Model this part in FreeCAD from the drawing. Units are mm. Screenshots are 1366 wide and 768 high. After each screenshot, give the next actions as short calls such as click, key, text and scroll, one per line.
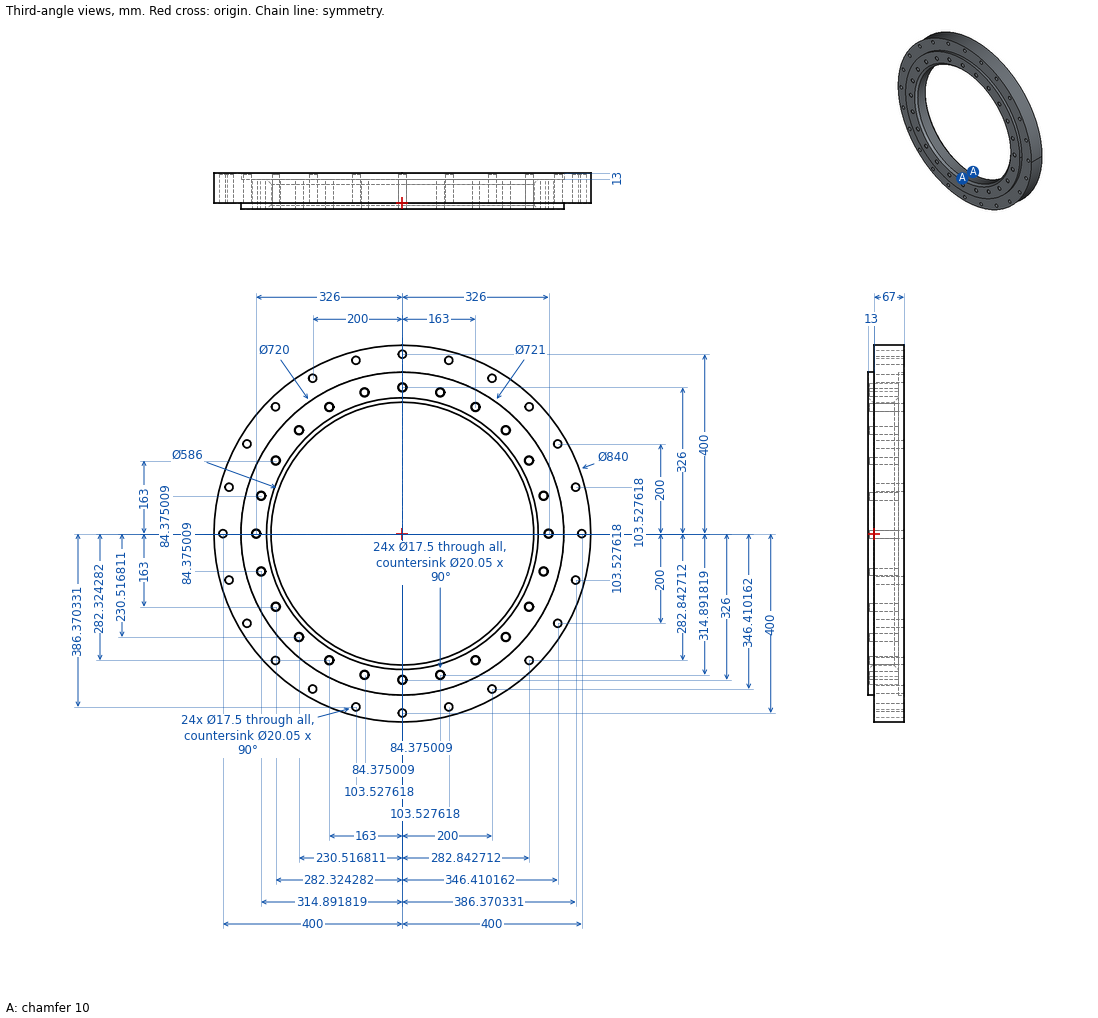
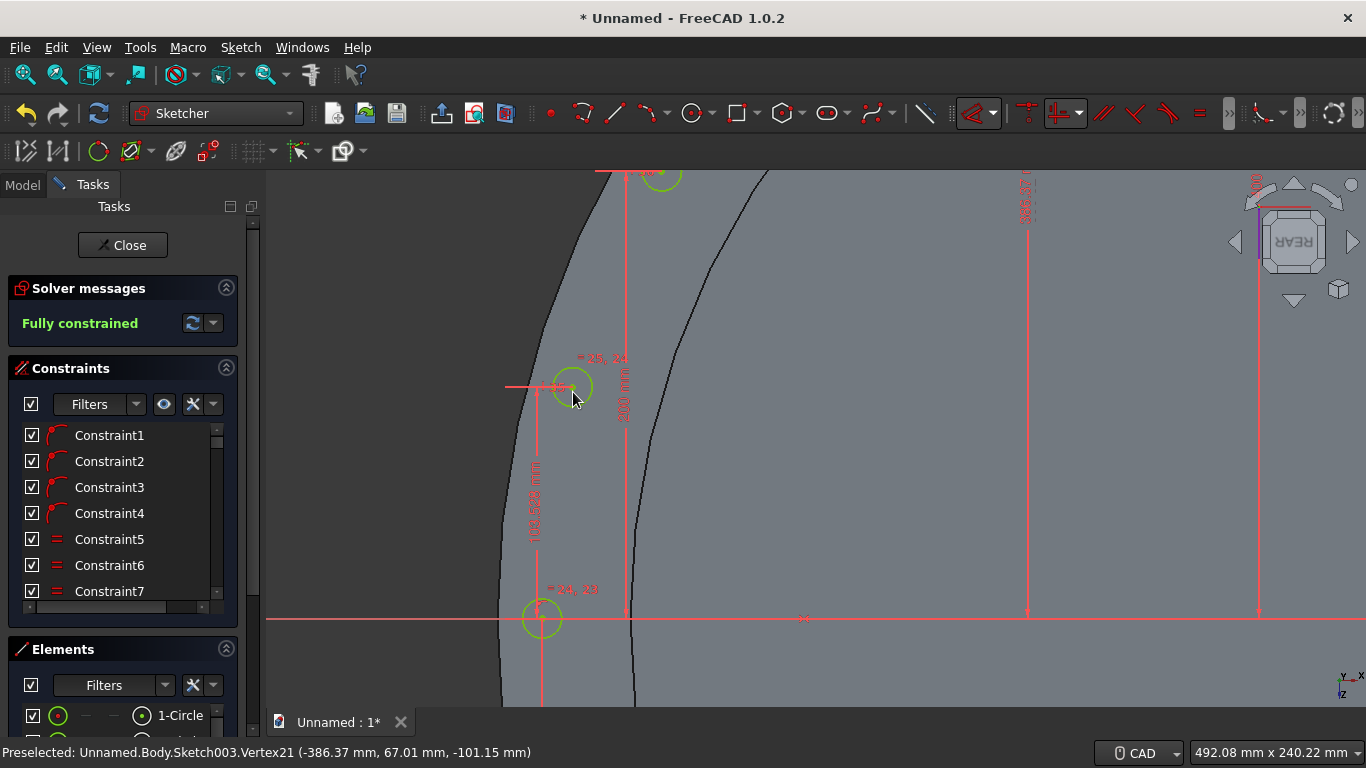
click(123, 245)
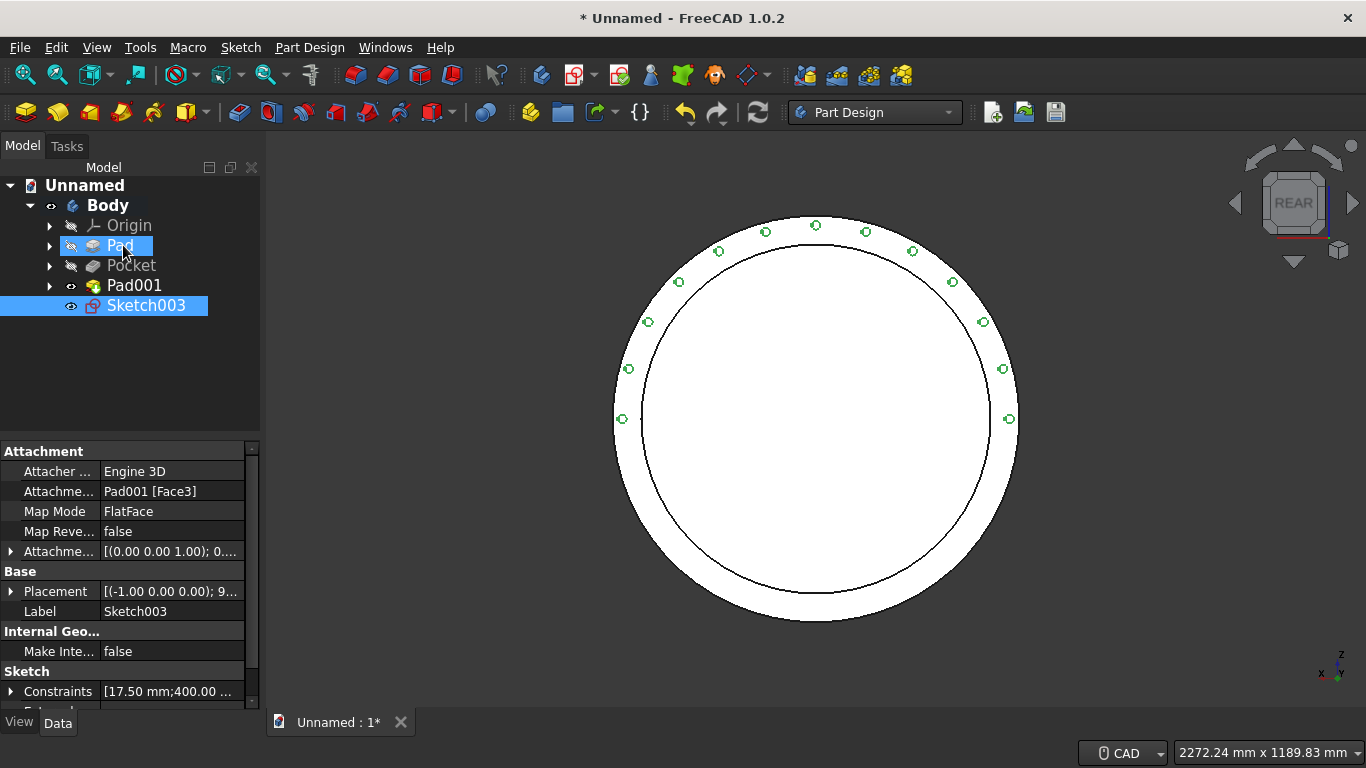
click(272, 112)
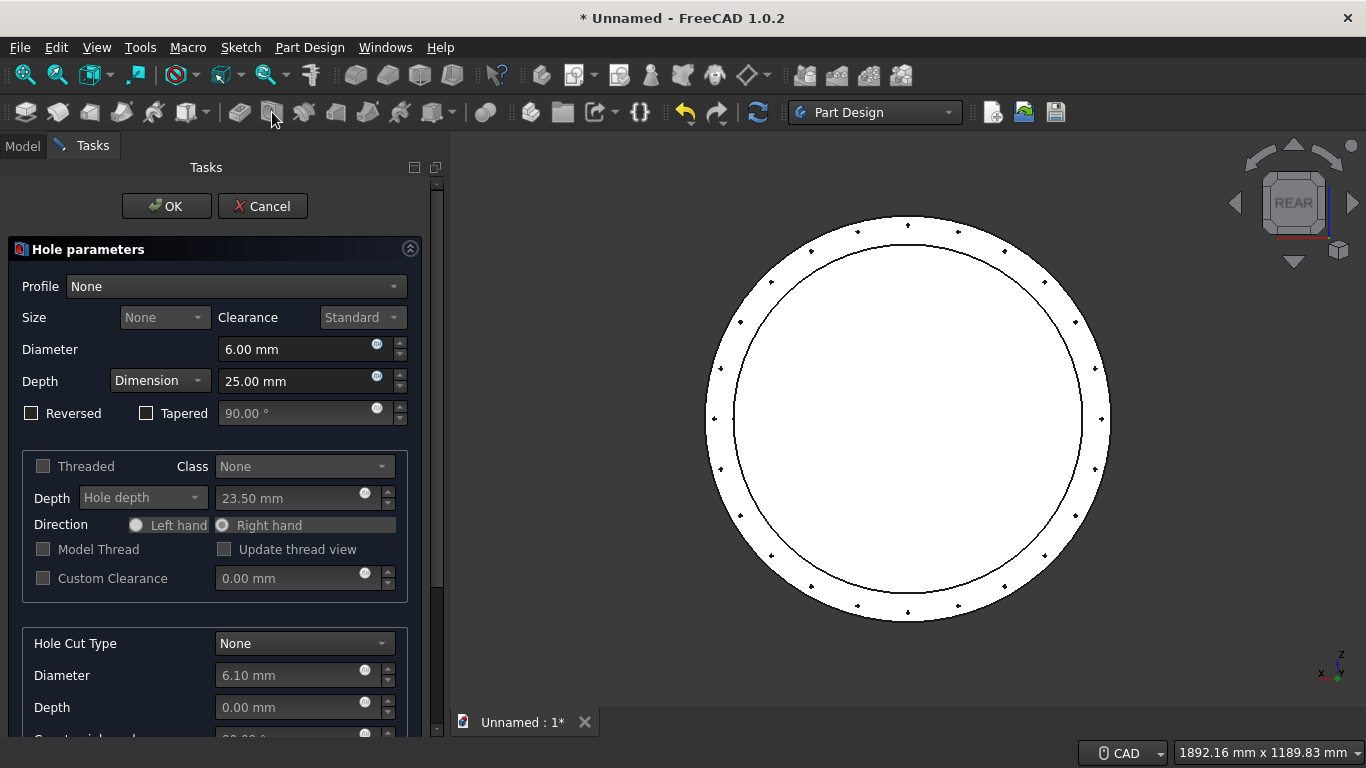
triple_click(305, 349)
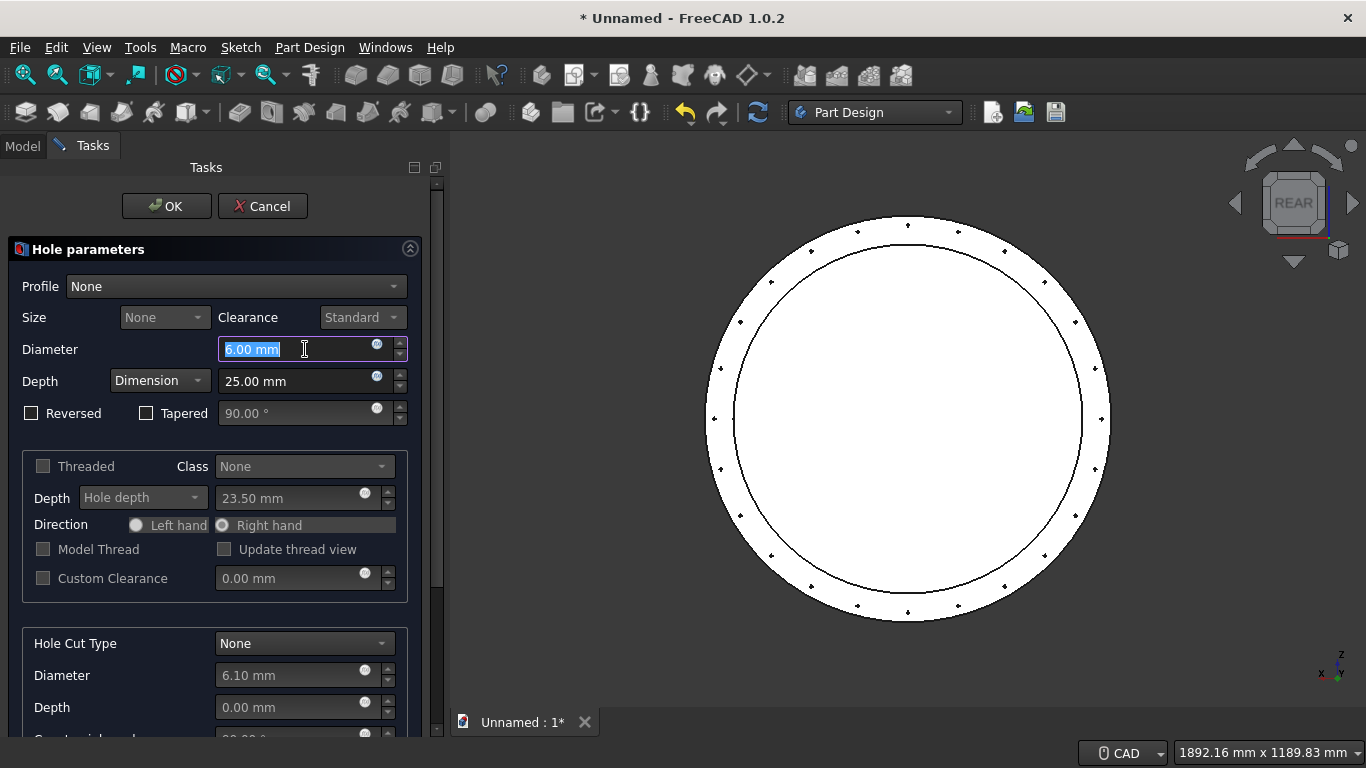
text(17.5)
key(Tab)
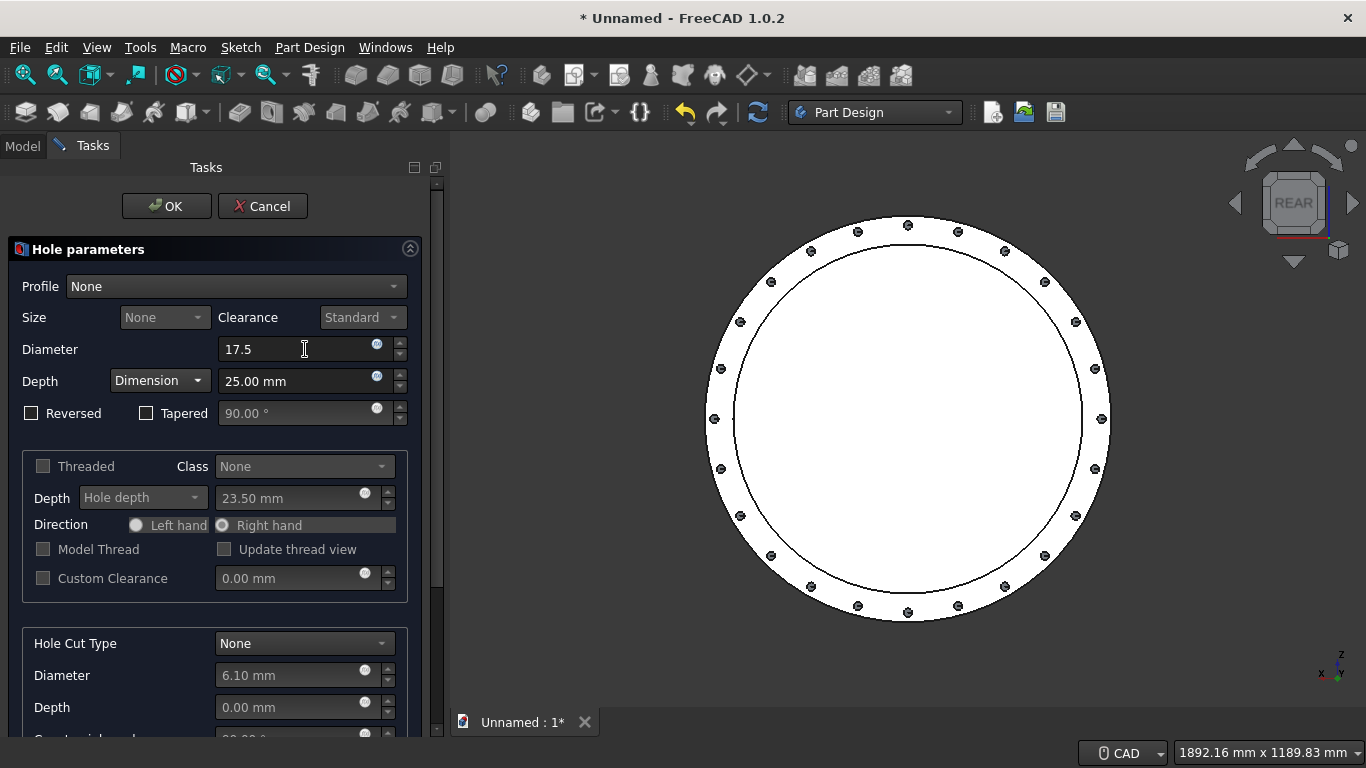
click(161, 380)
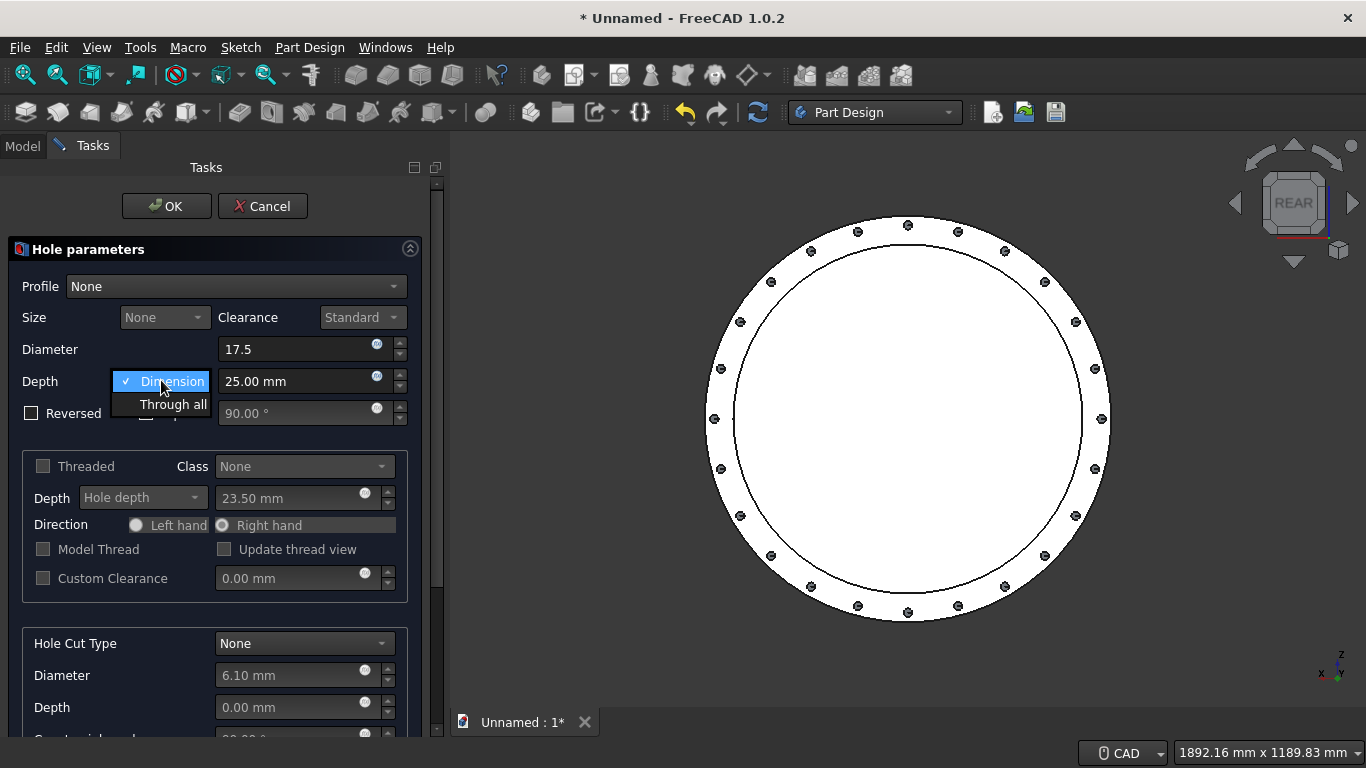
click(160, 404)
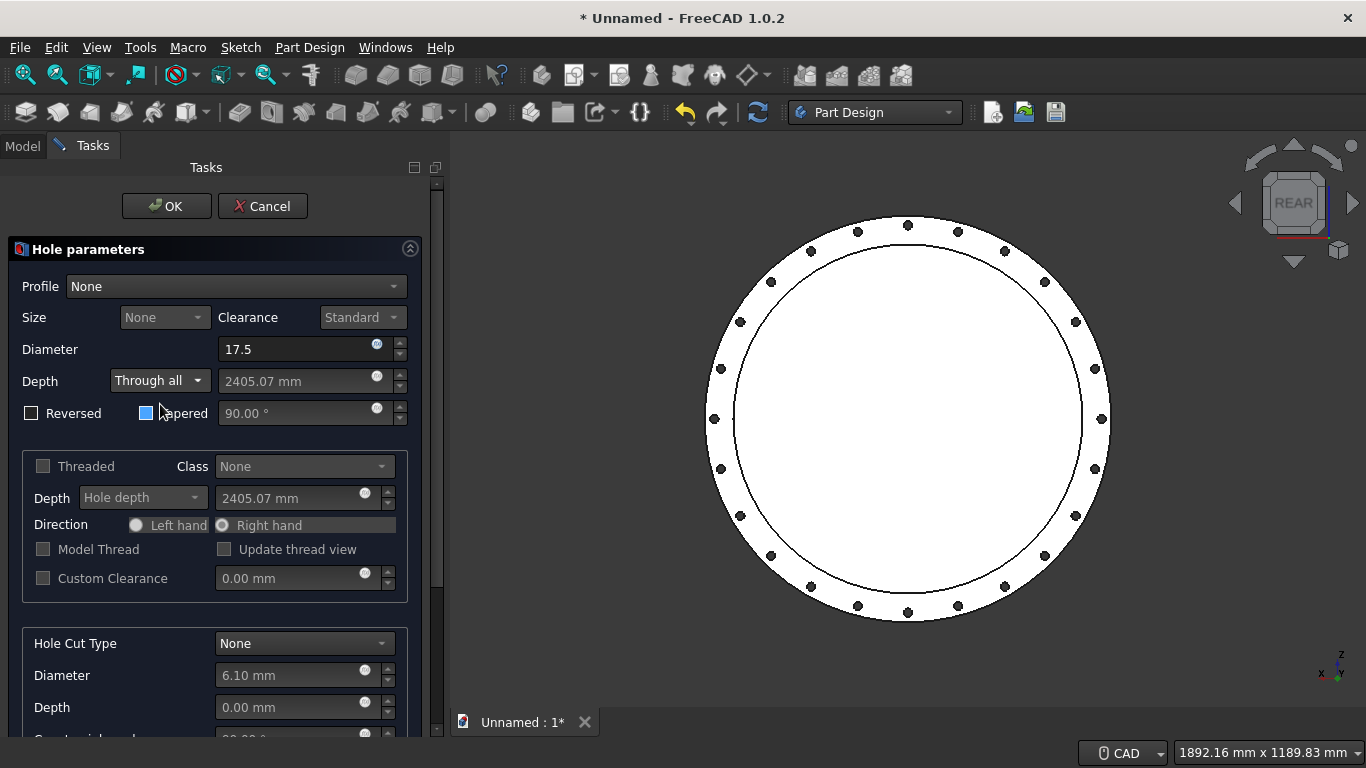
click(306, 644)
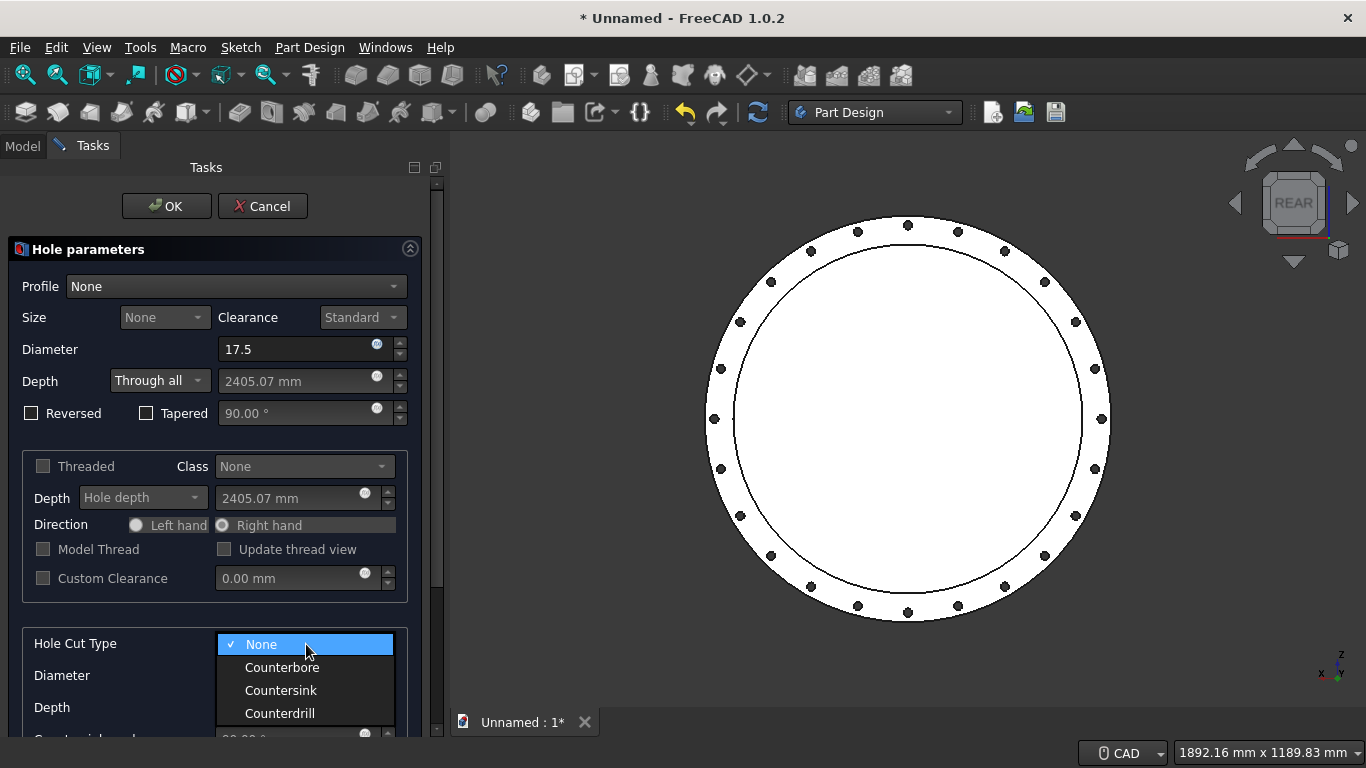
click(304, 690)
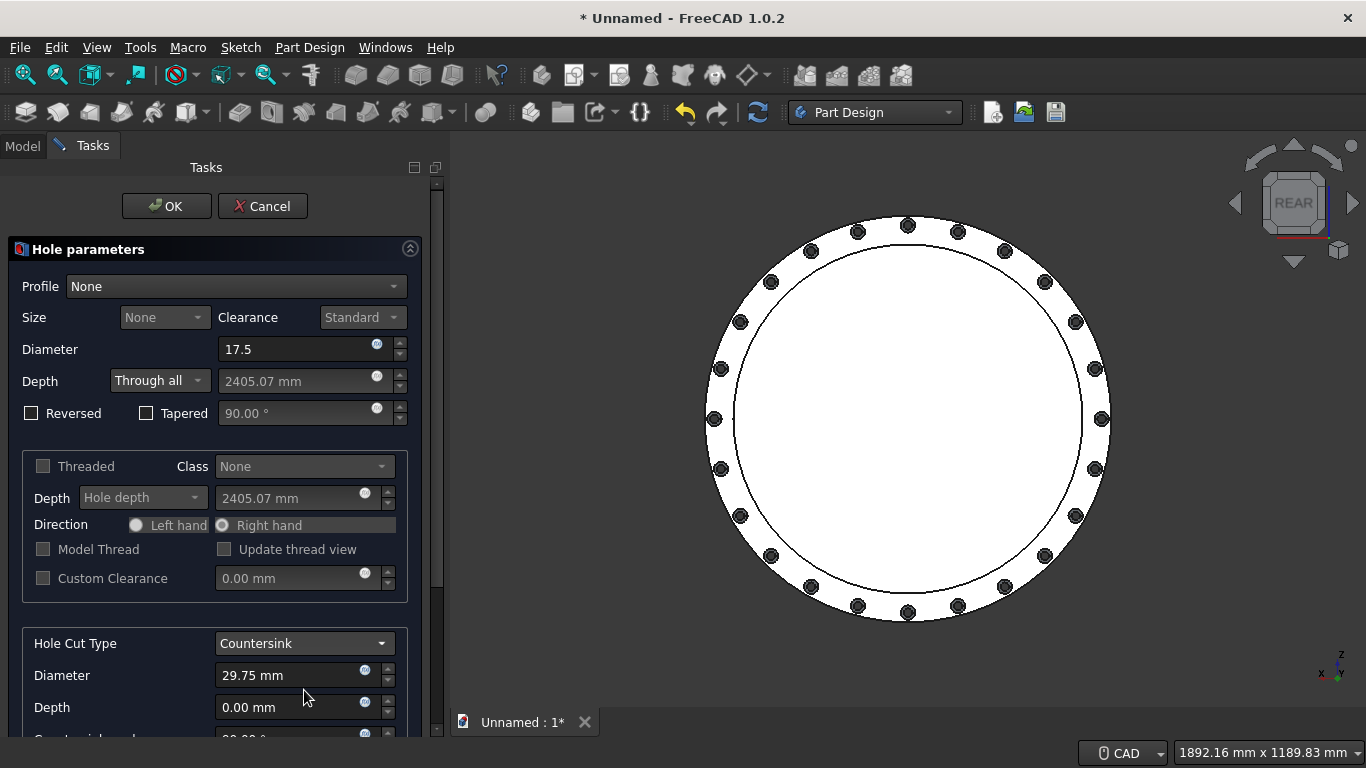
triple_click(298, 675)